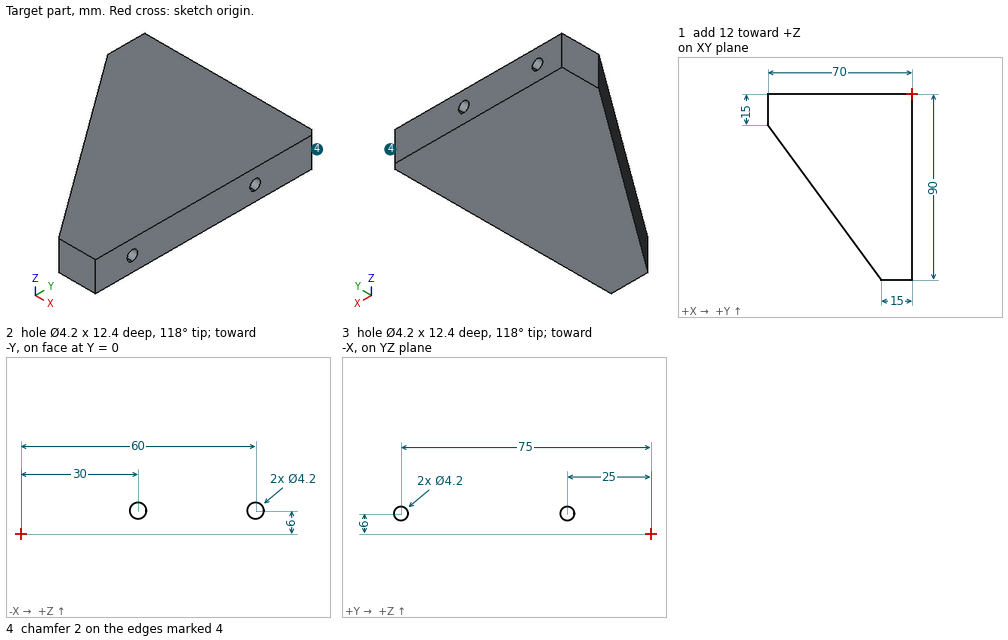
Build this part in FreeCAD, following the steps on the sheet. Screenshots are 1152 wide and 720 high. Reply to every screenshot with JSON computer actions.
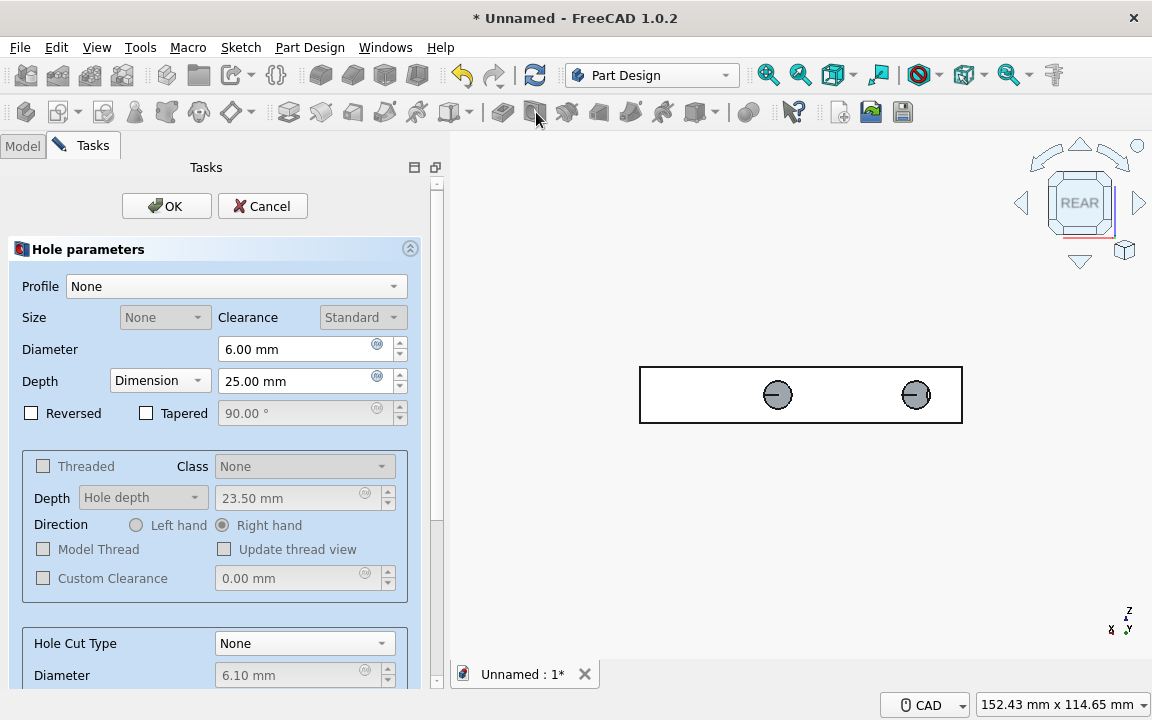
{"action": "triple_click", "coordinate": [305, 349]}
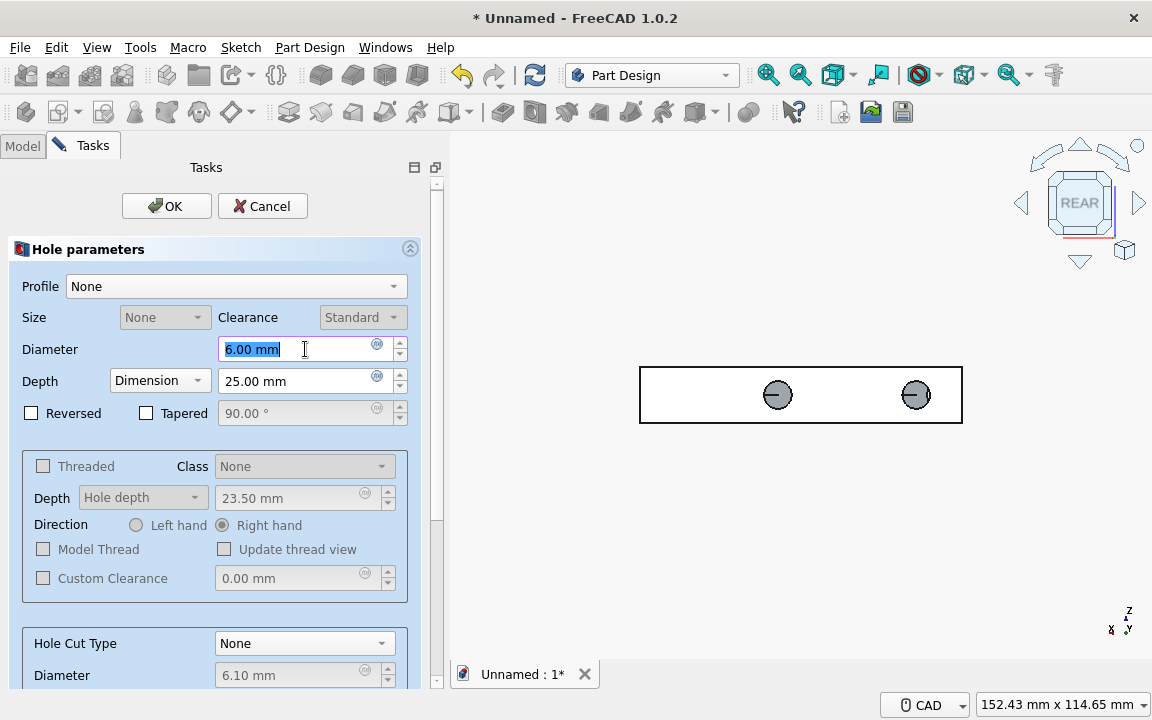
{"action": "type", "text": "4.2"}
{"action": "key", "text": "Tab"}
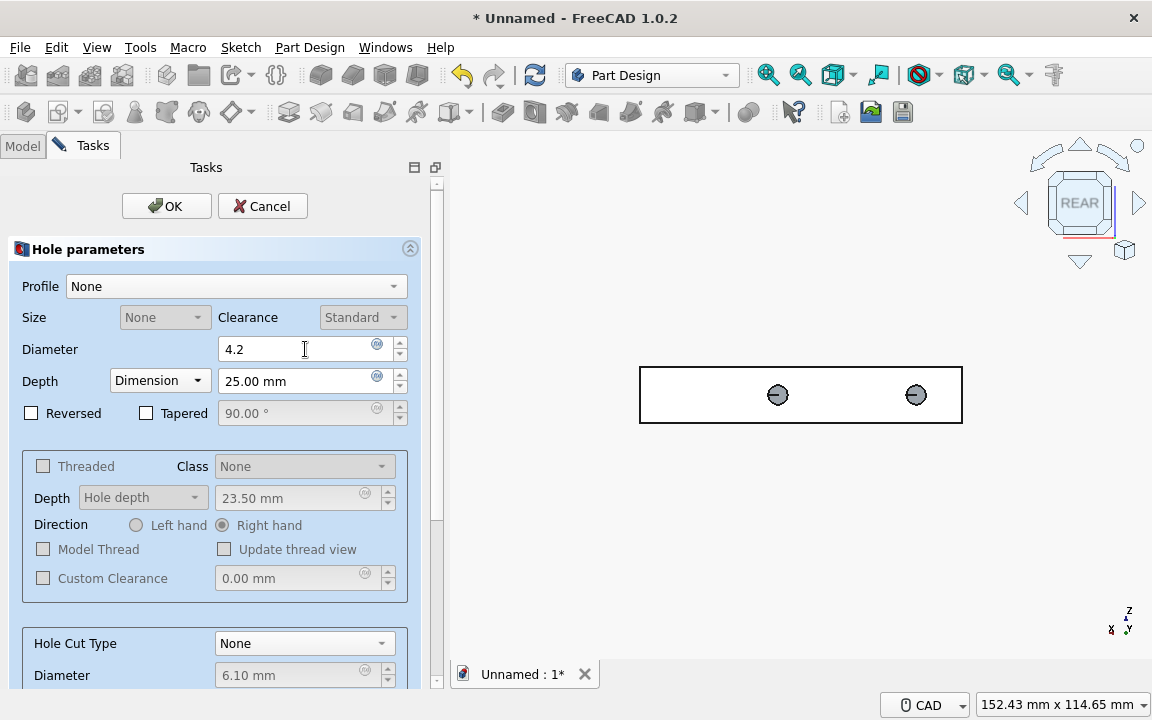
{"action": "triple_click", "coordinate": [305, 381]}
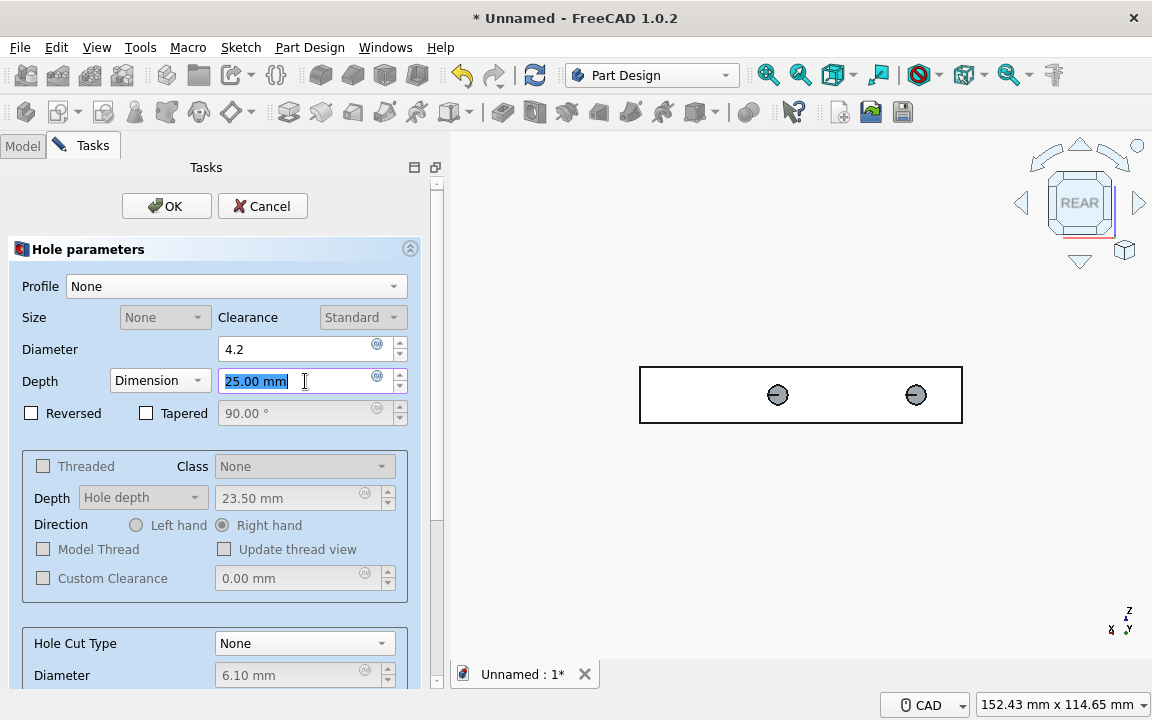
{"action": "type", "text": "12.4"}
{"action": "key", "text": "Tab"}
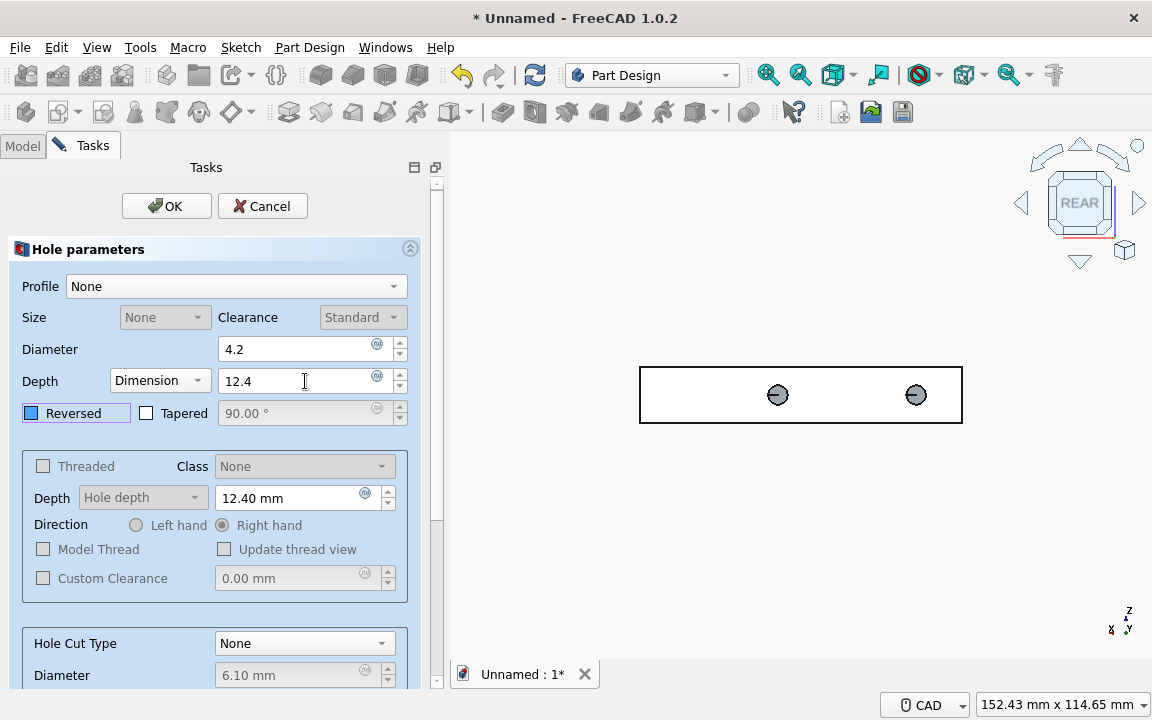
{"action": "left_click", "coordinate": [167, 206]}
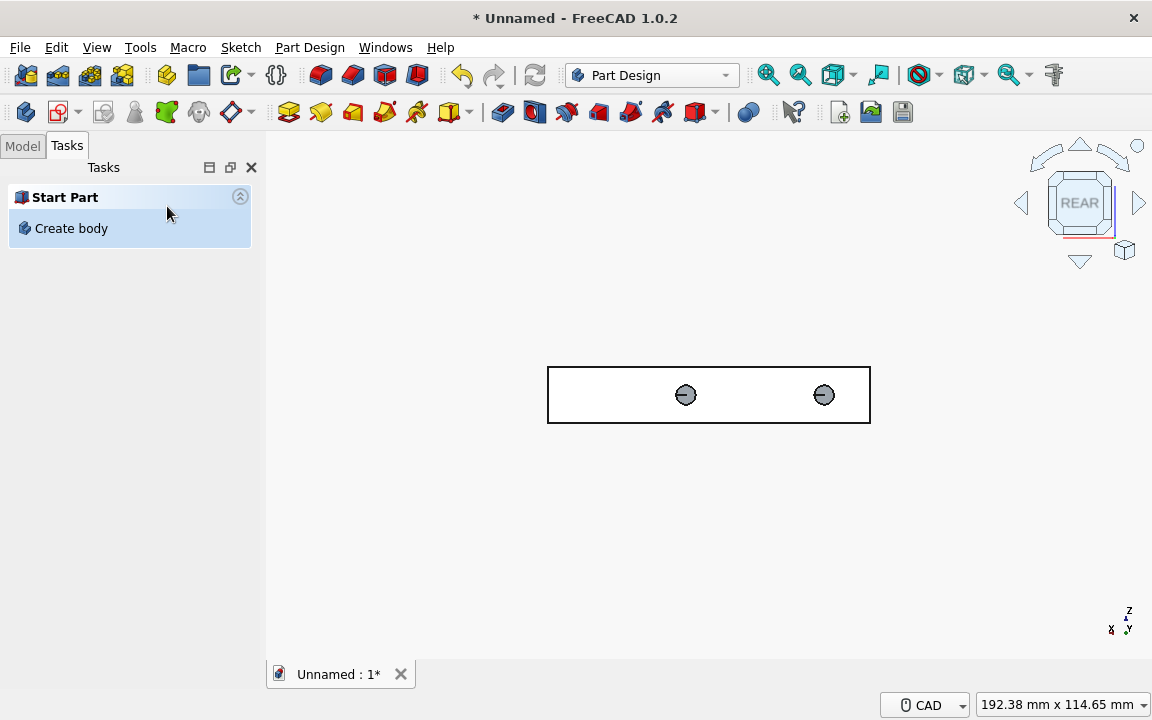
{"action": "left_click", "coordinate": [770, 76]}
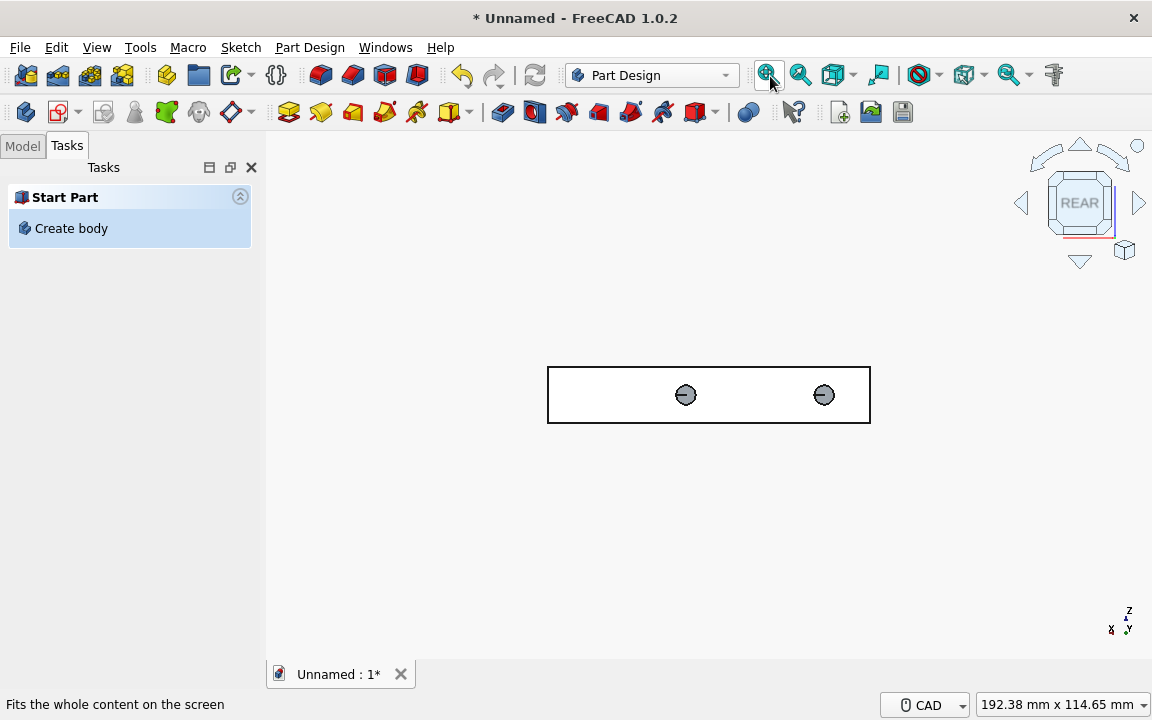
{"action": "left_click", "coordinate": [58, 112]}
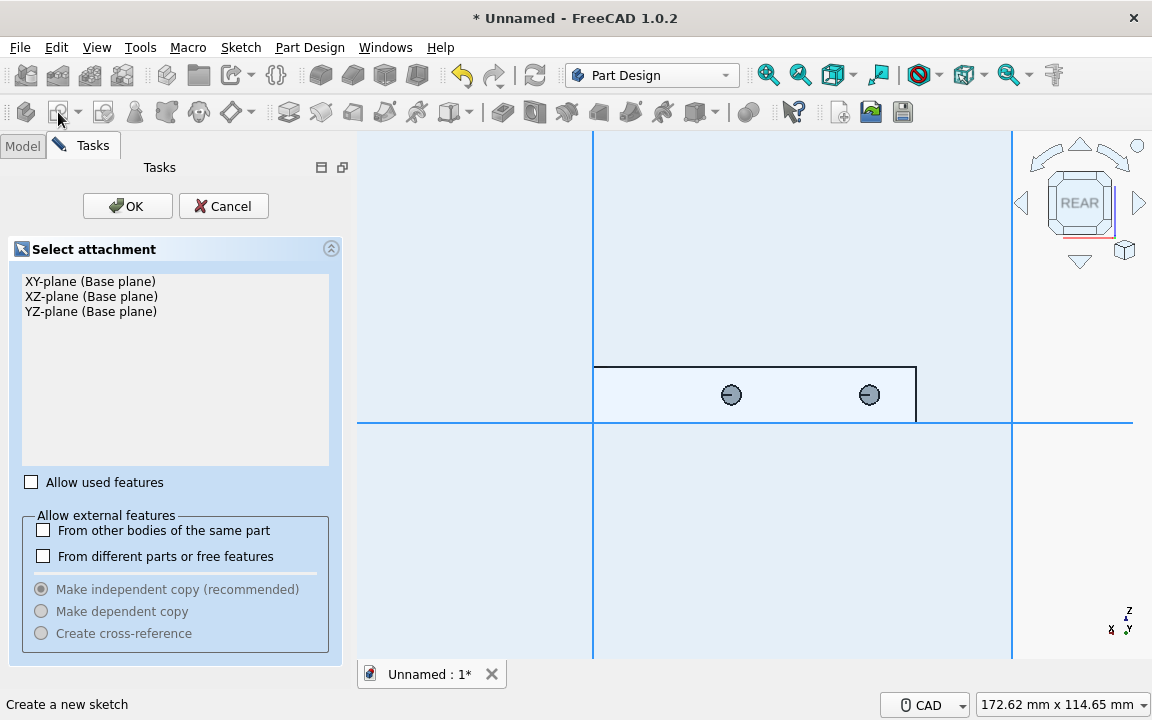
{"action": "left_click", "coordinate": [82, 312]}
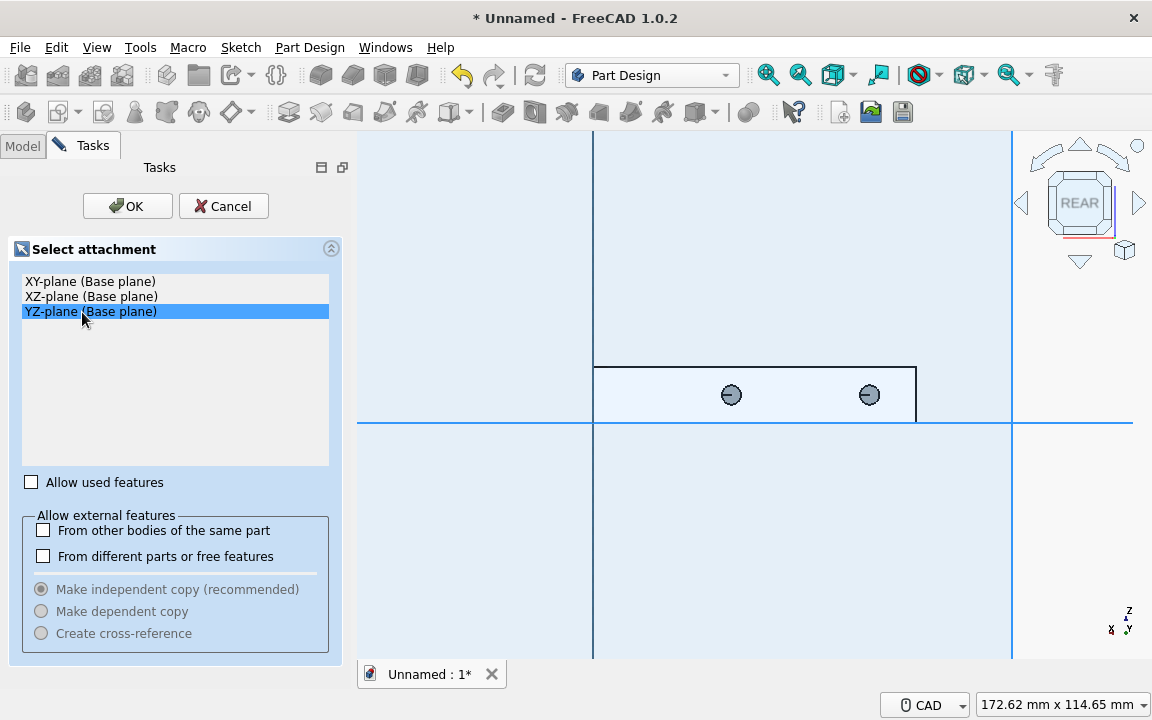
{"action": "left_click", "coordinate": [128, 206]}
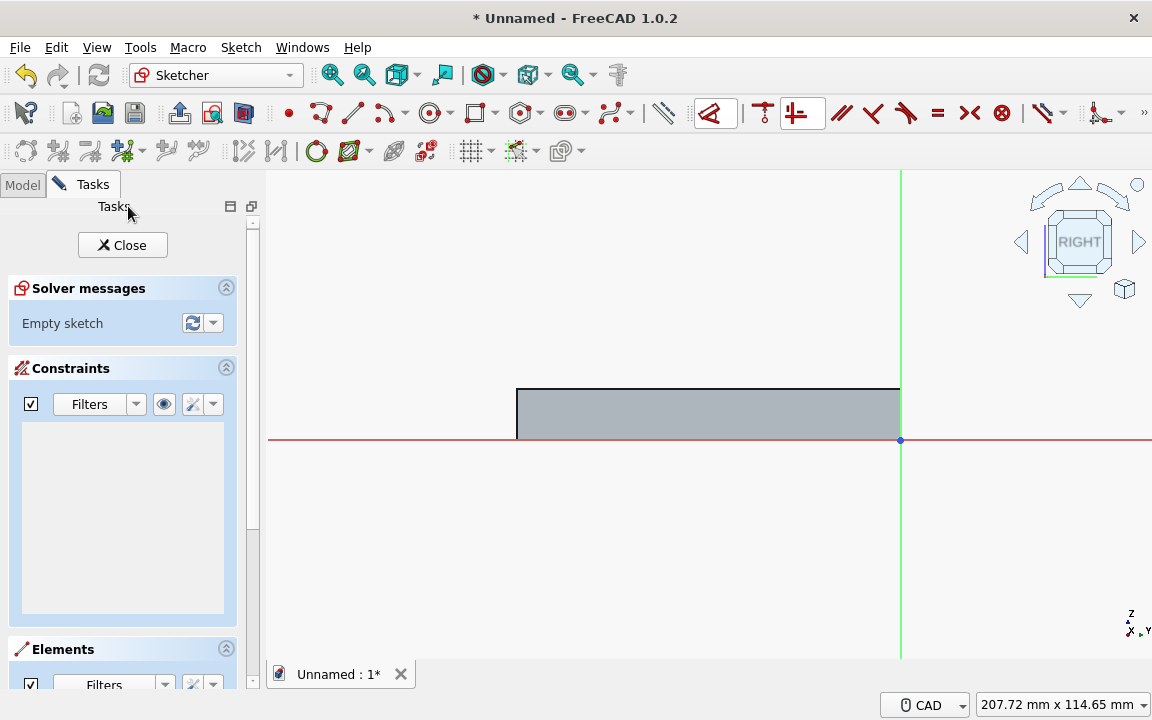
{"action": "scroll", "coordinate": [932, 440], "scroll_direction": "up", "scroll_amount": 2}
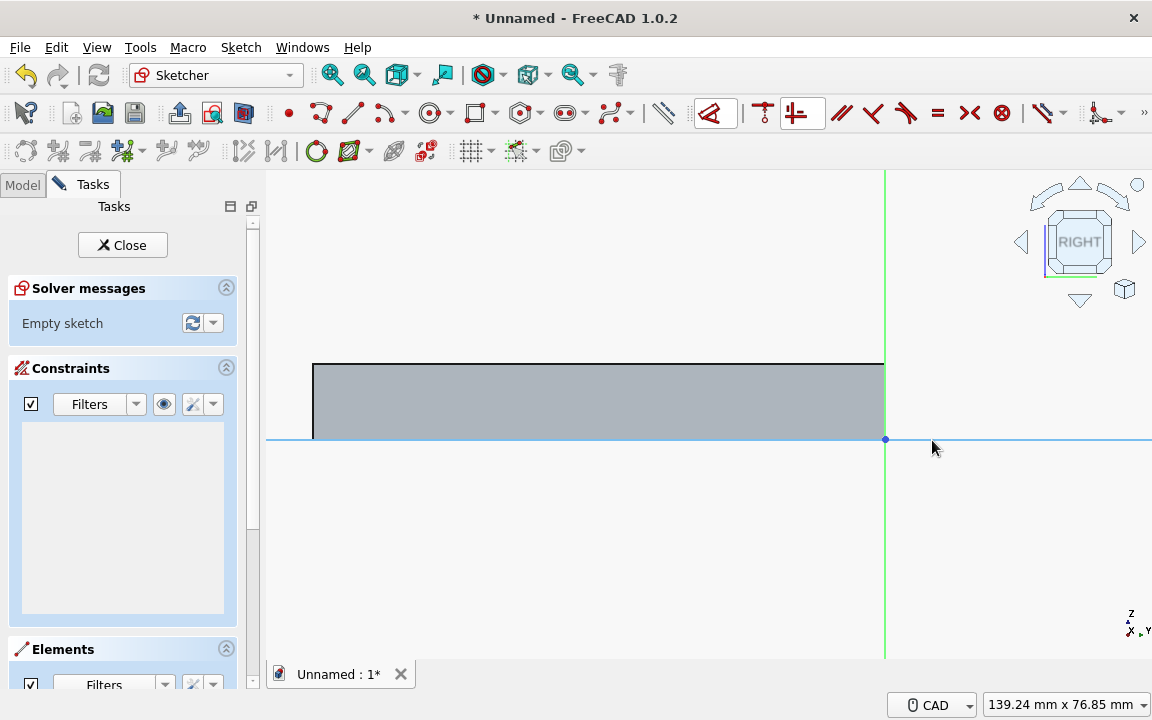
{"action": "left_click", "coordinate": [430, 114]}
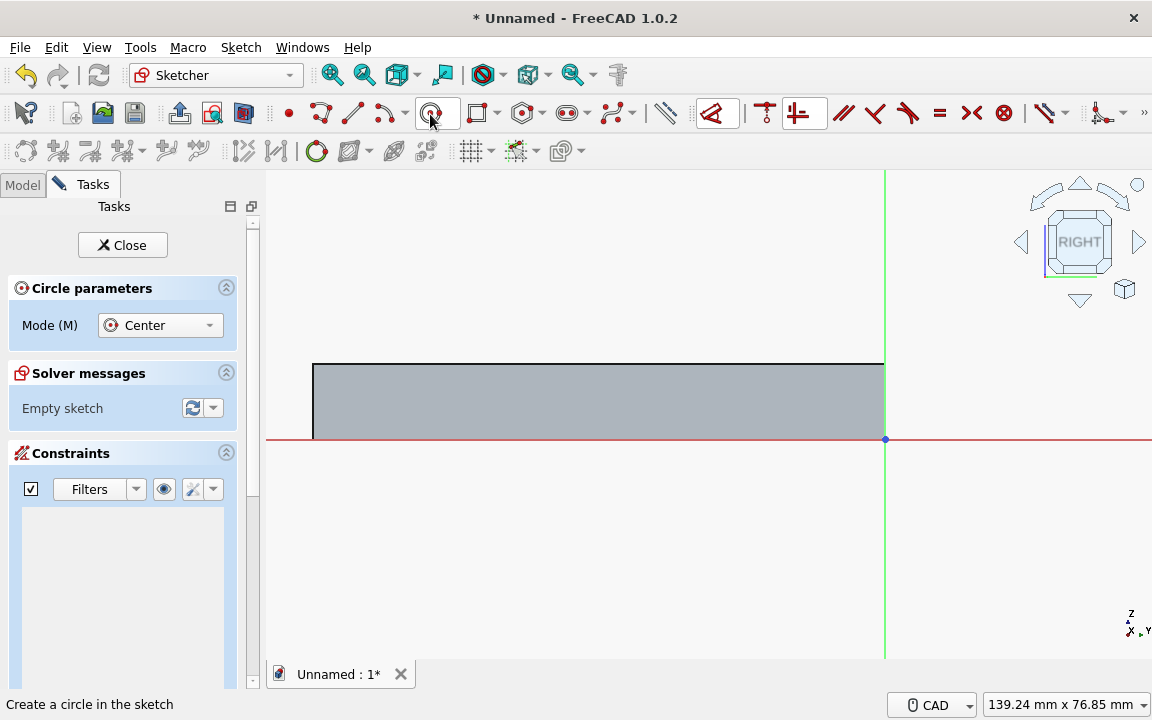
{"action": "scroll", "coordinate": [408, 402], "scroll_direction": "up", "scroll_amount": 3}